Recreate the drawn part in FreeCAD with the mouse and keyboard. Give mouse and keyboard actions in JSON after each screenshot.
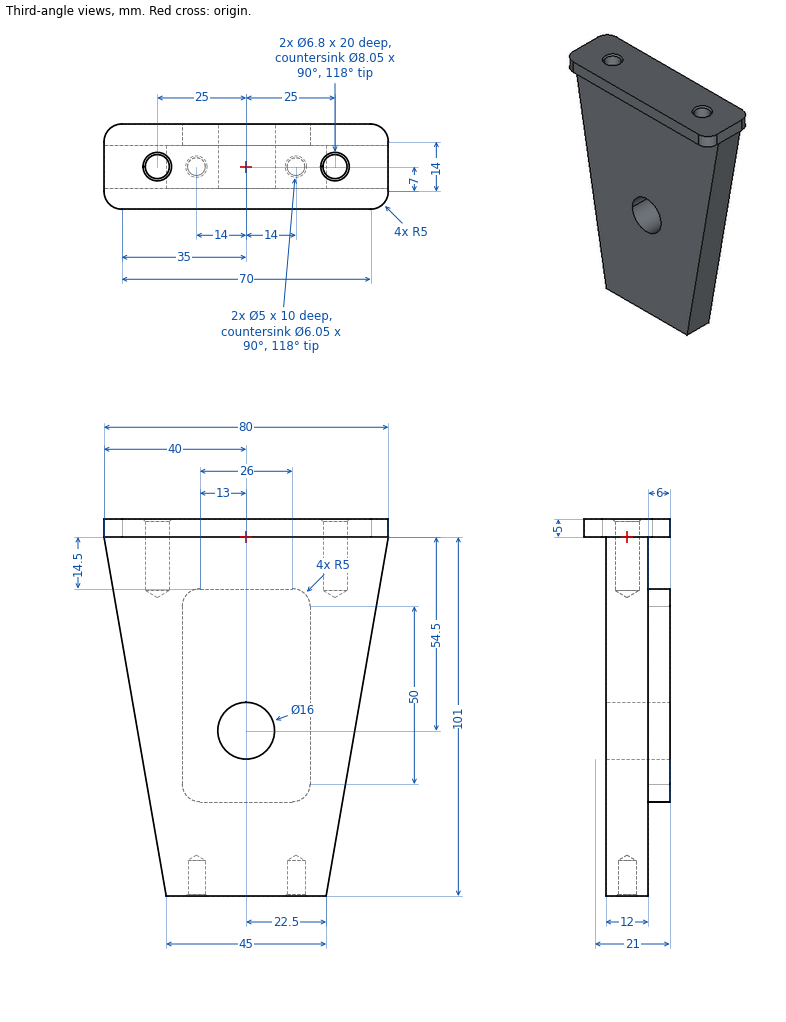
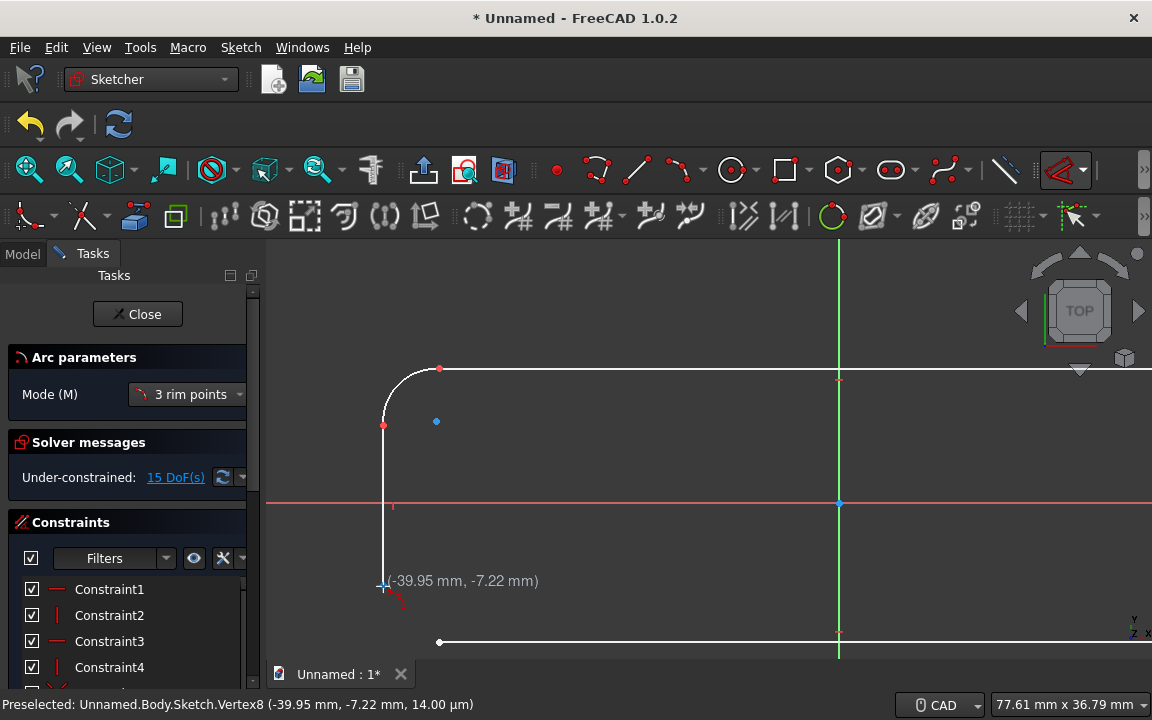
{"action": "scroll", "coordinate": [399, 383], "scroll_direction": "down", "scroll_amount": 3}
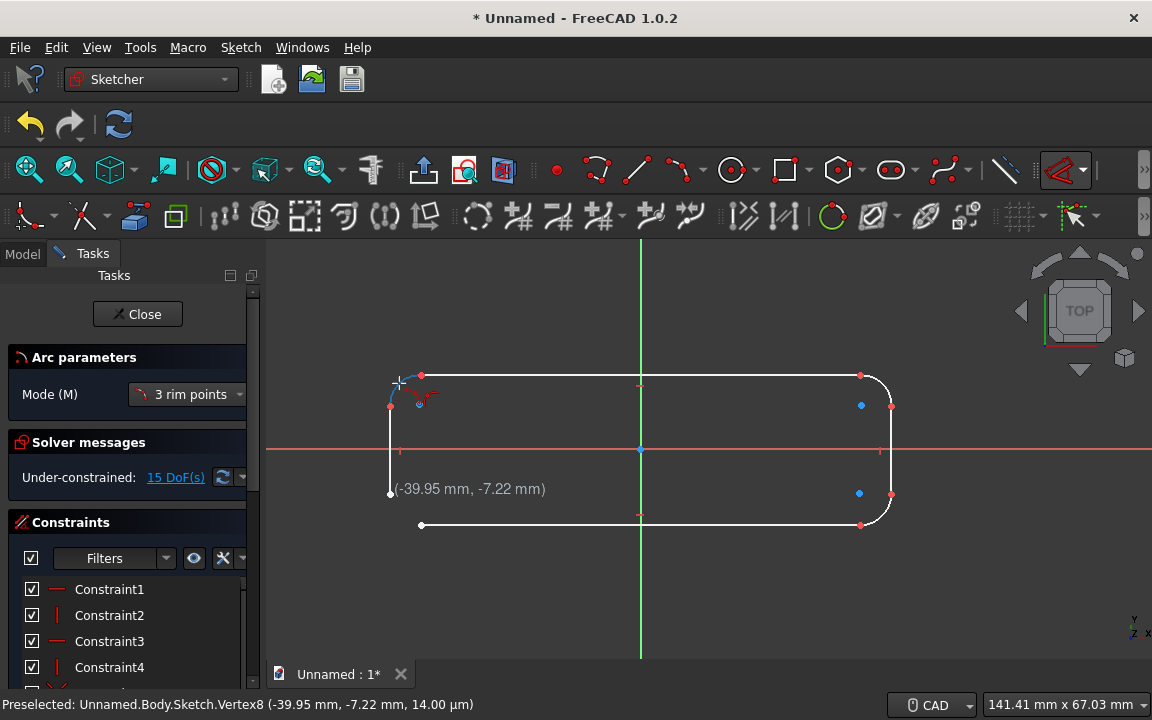
{"action": "left_click", "coordinate": [421, 525]}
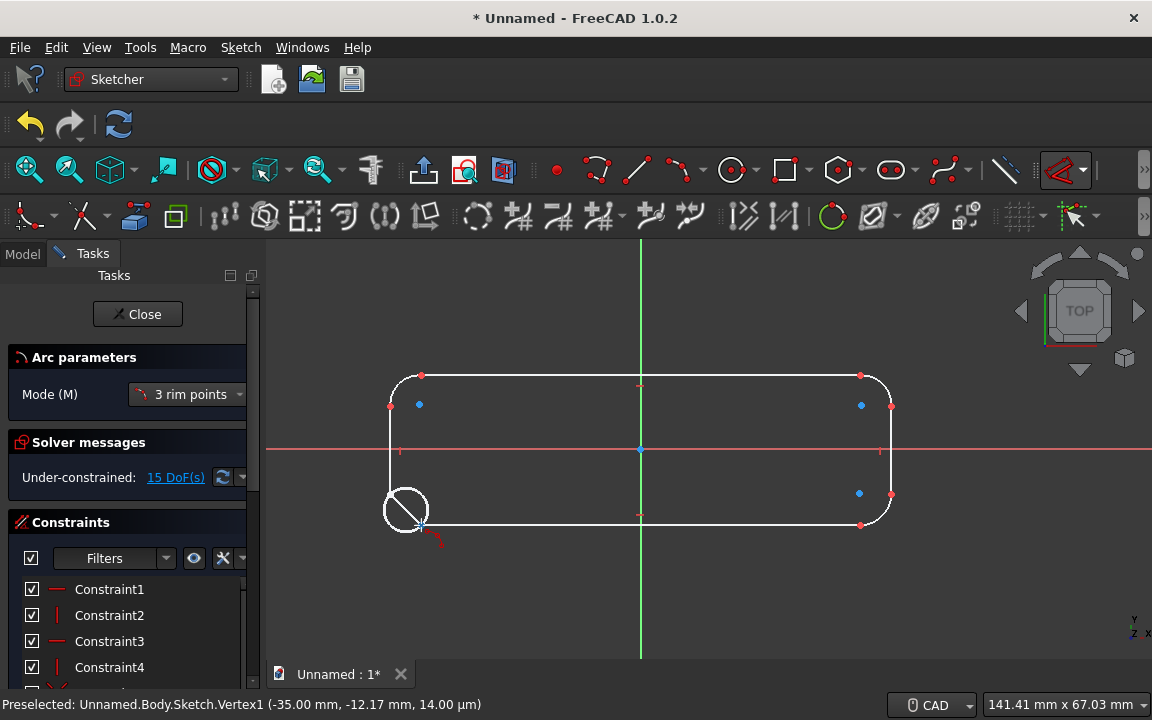
{"action": "scroll", "coordinate": [399, 515], "scroll_direction": "up", "scroll_amount": 3}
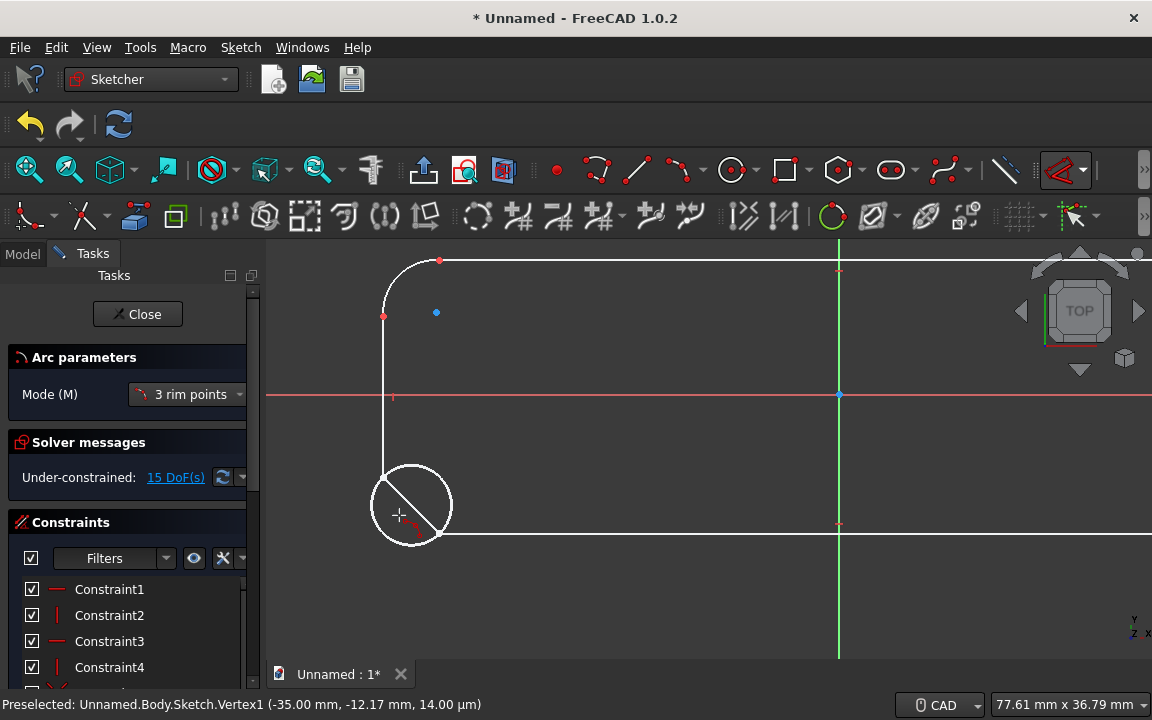
{"action": "left_click", "coordinate": [399, 515]}
{"action": "key", "text": "Escape"}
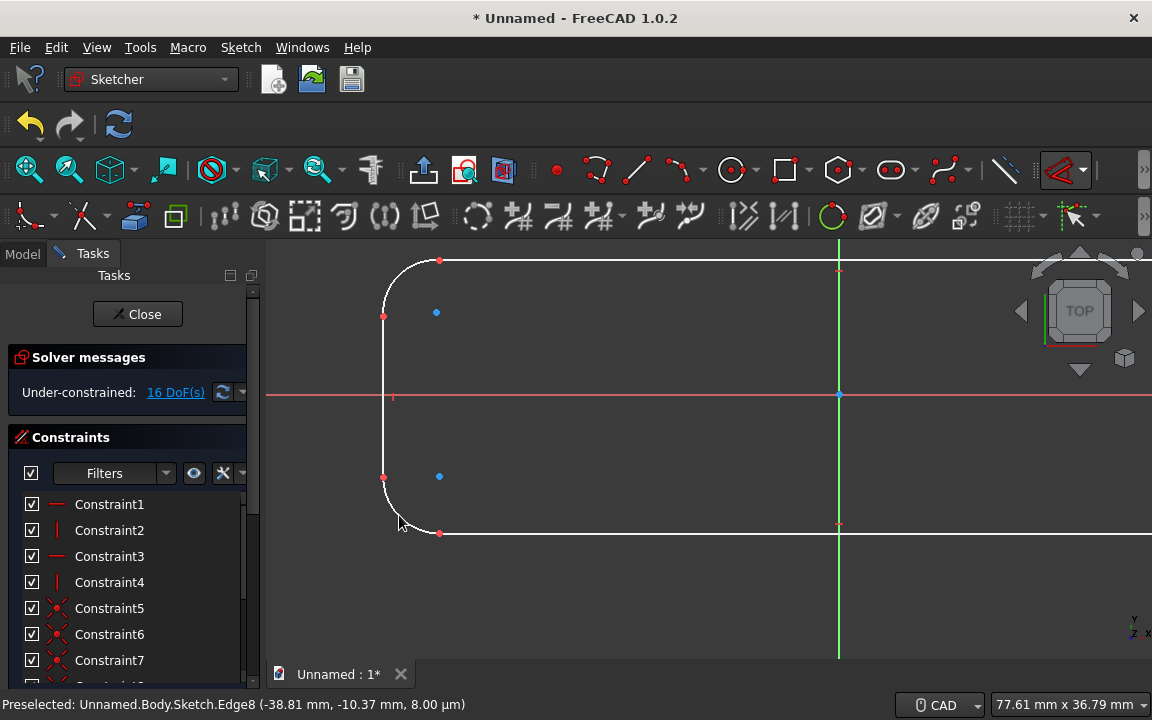
{"action": "left_click", "coordinate": [680, 534]}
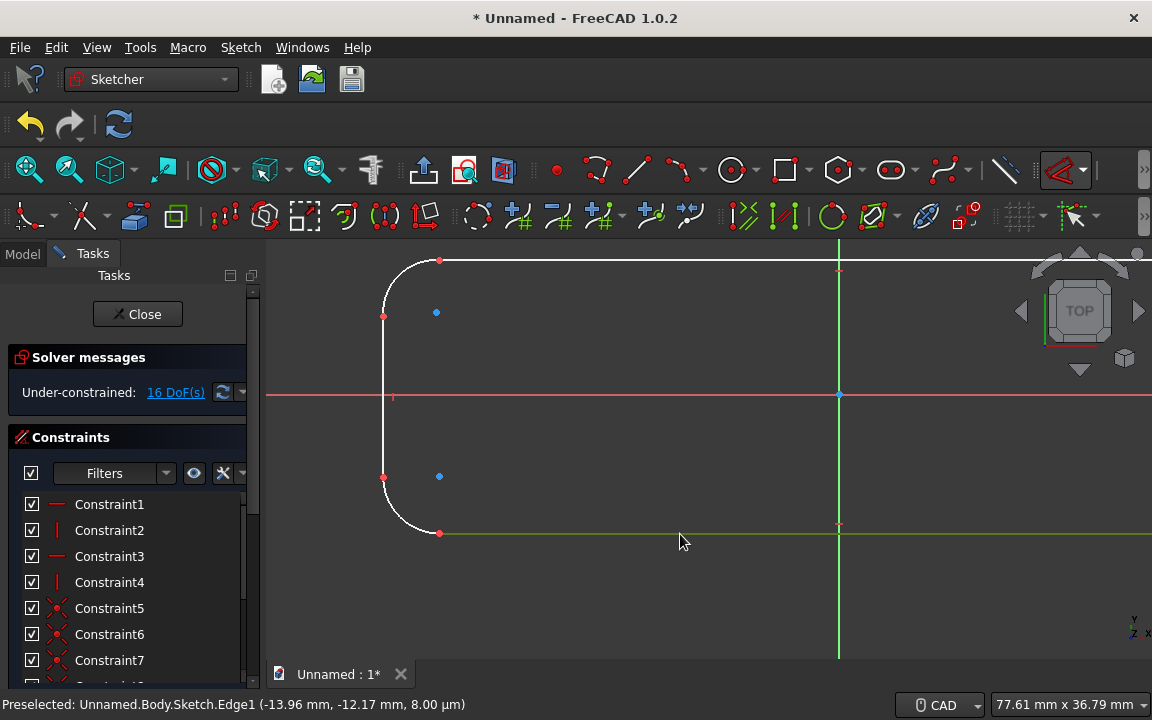
{"action": "scroll", "coordinate": [399, 515], "scroll_direction": "down", "scroll_amount": 3}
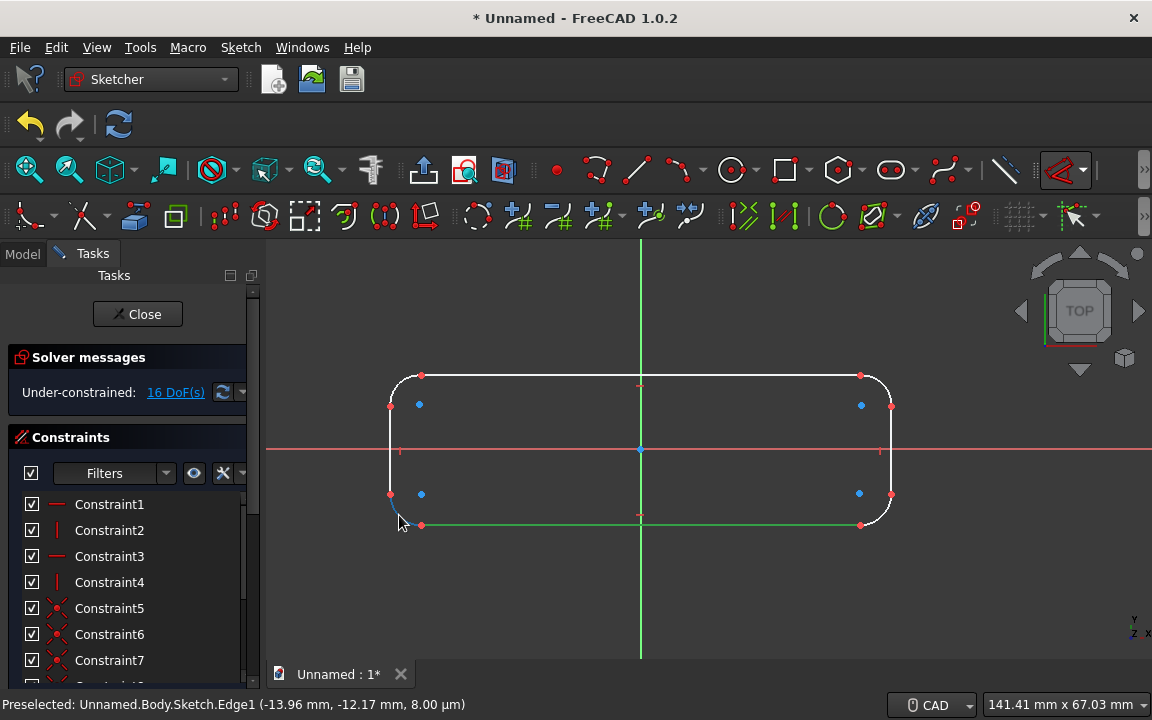
{"action": "left_click", "coordinate": [874, 522]}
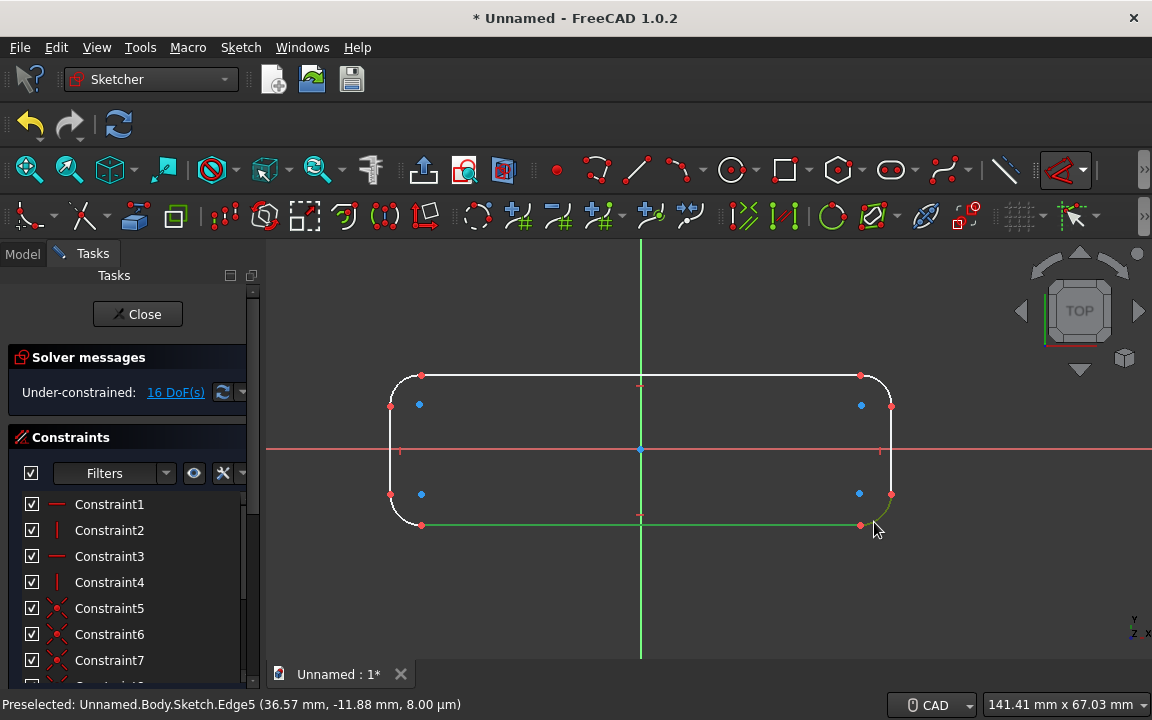
{"action": "key", "text": "t"}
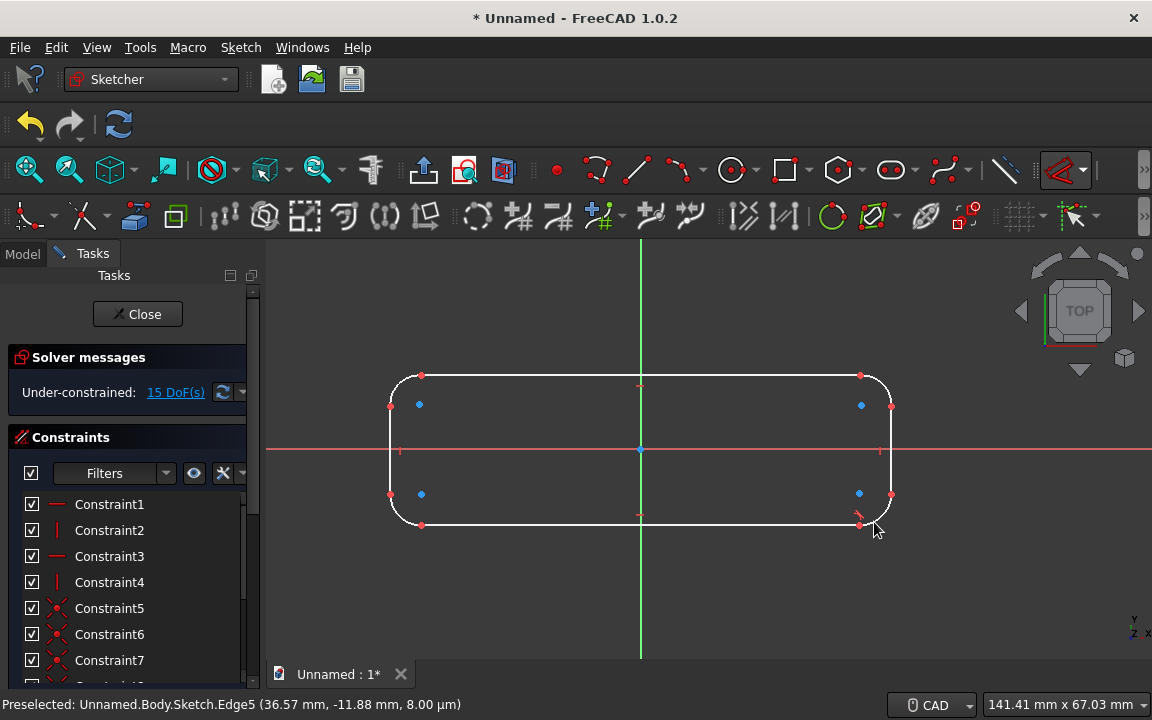
{"action": "left_click", "coordinate": [553, 525]}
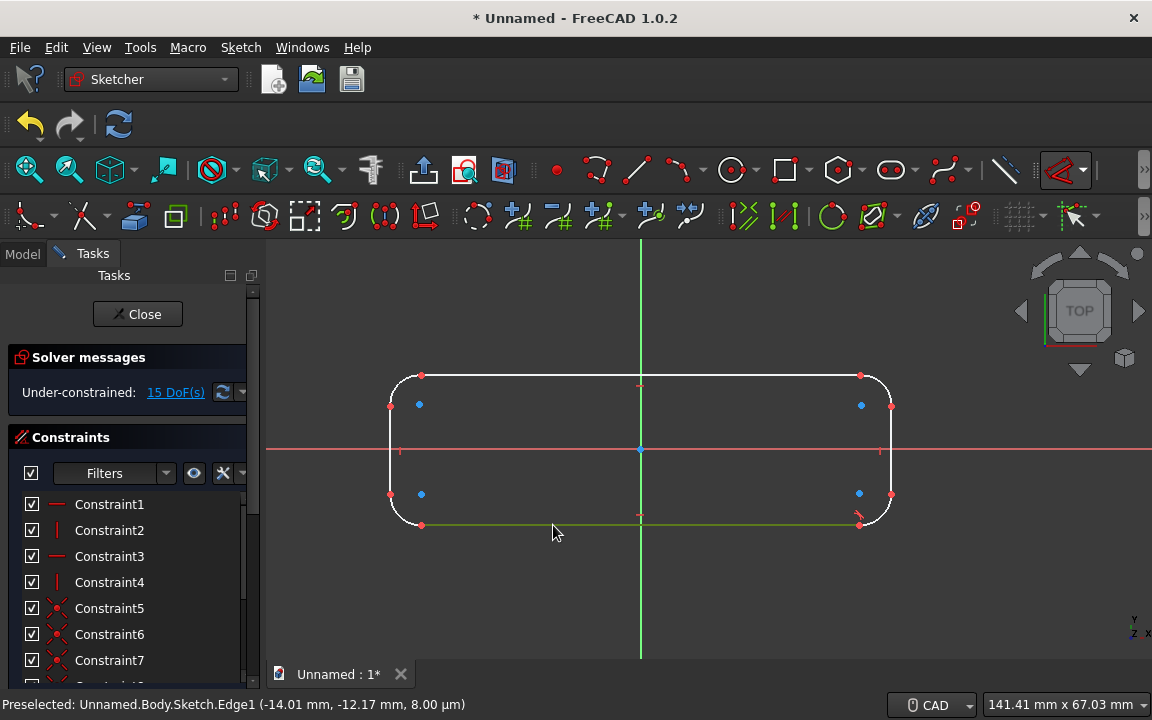
{"action": "left_click", "coordinate": [394, 509]}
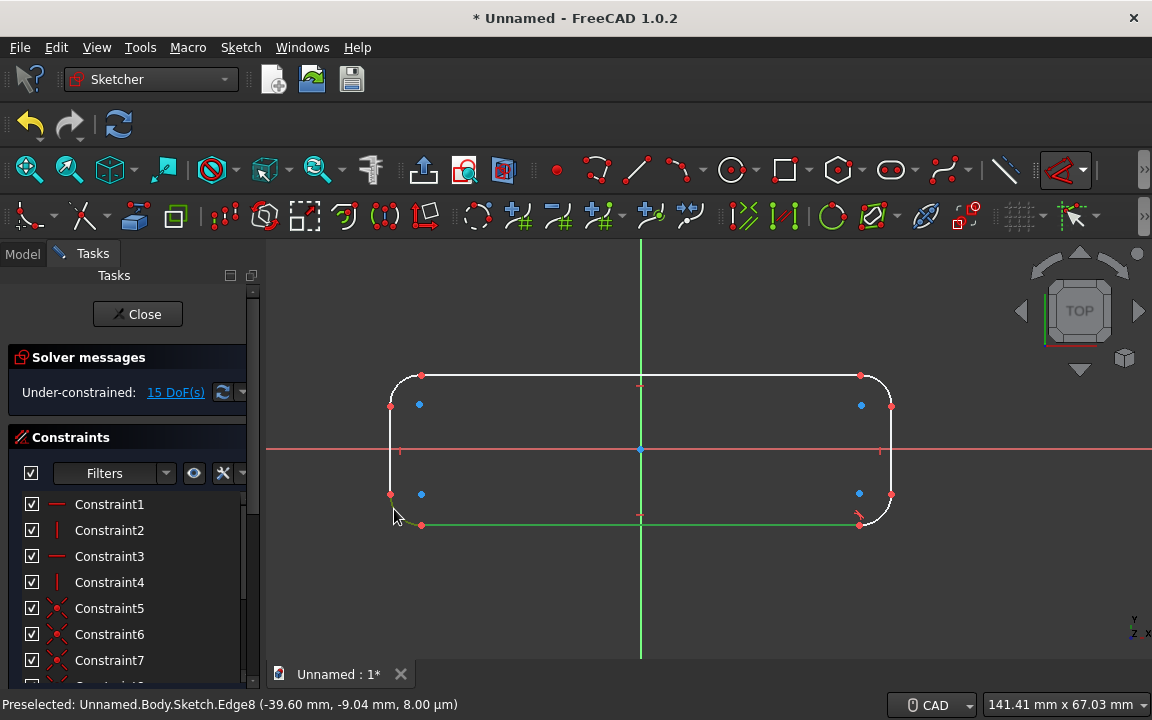
{"action": "key", "text": "t"}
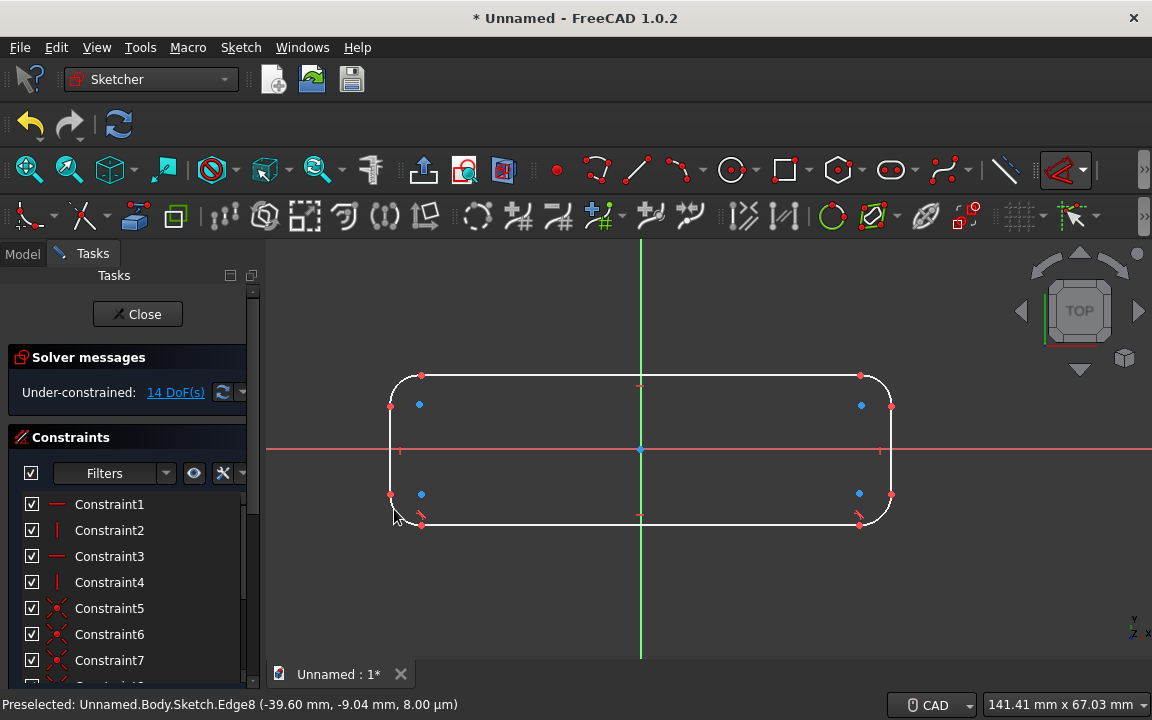
{"action": "left_click", "coordinate": [891, 468]}